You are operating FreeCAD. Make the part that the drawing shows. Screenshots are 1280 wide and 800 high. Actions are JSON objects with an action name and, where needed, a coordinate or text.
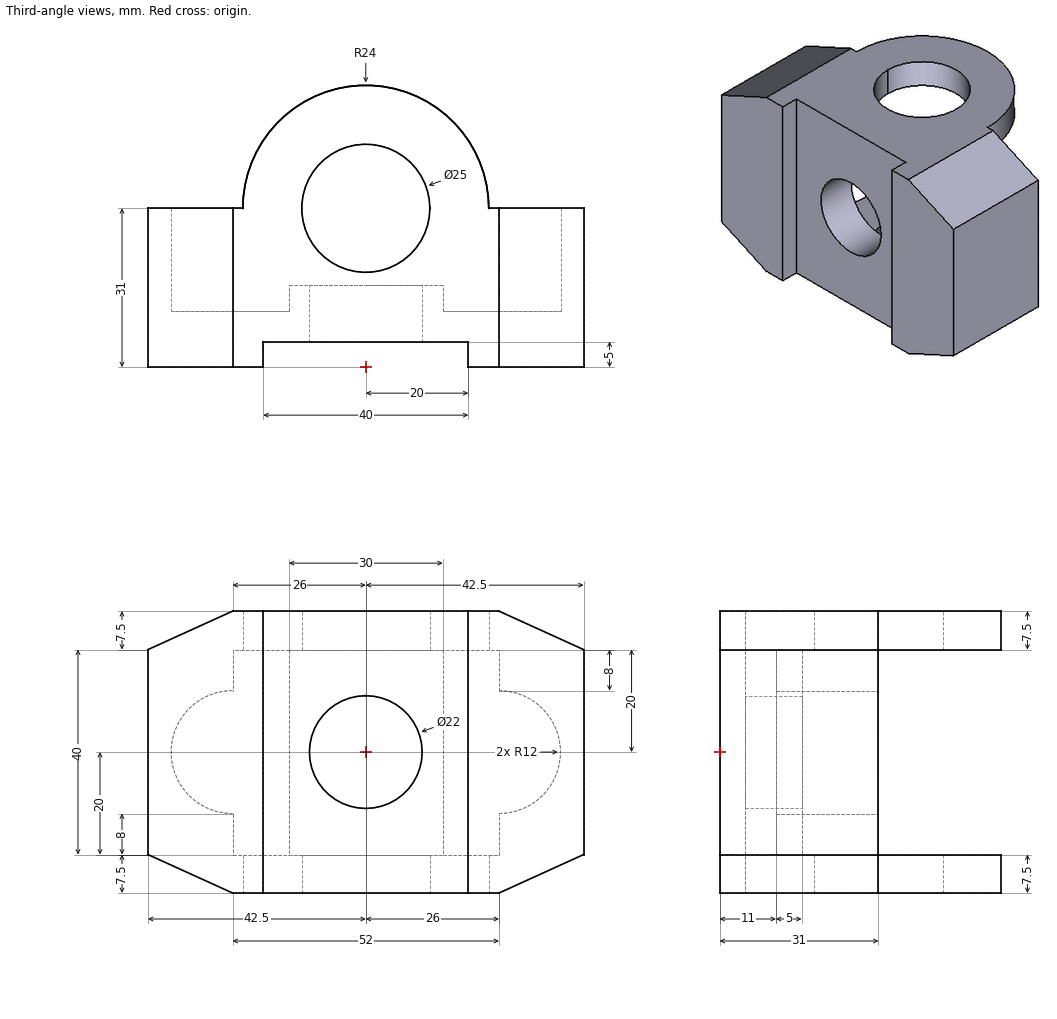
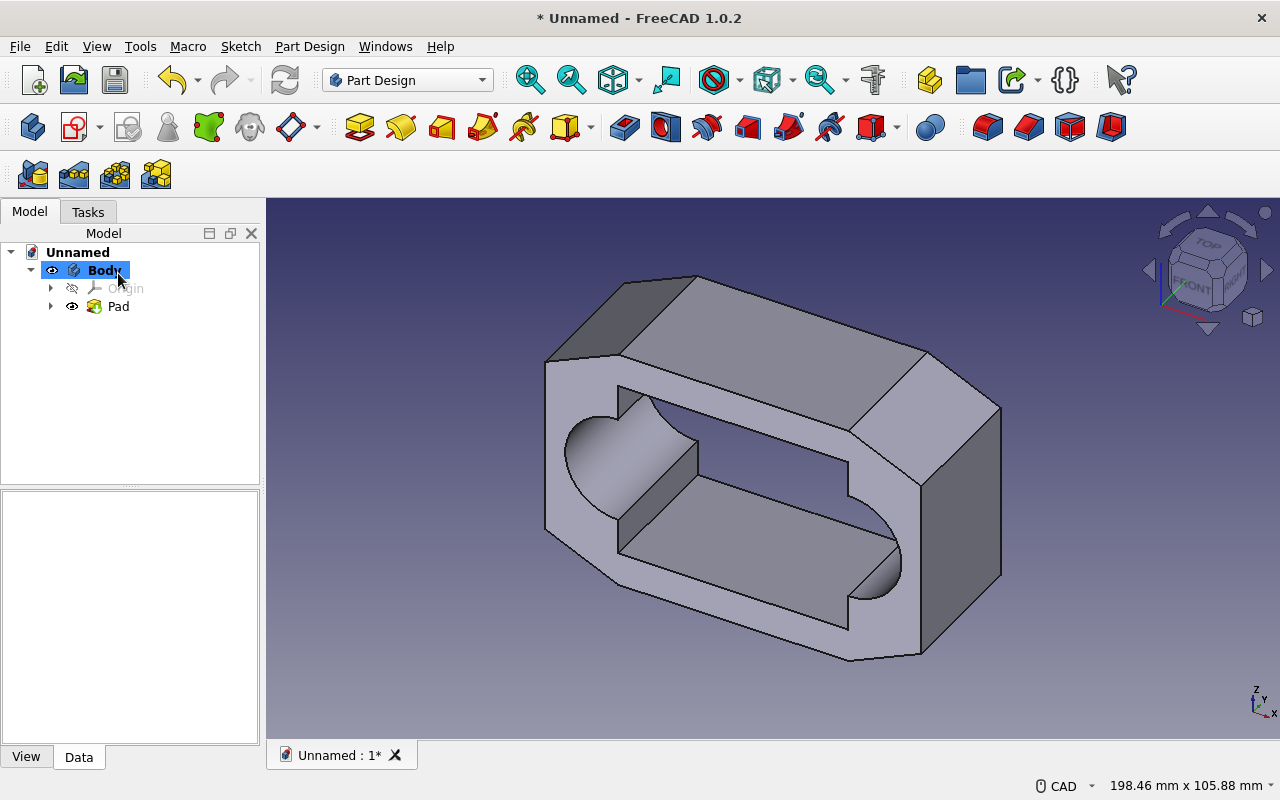
{"action": "left_click", "coordinate": [806, 363]}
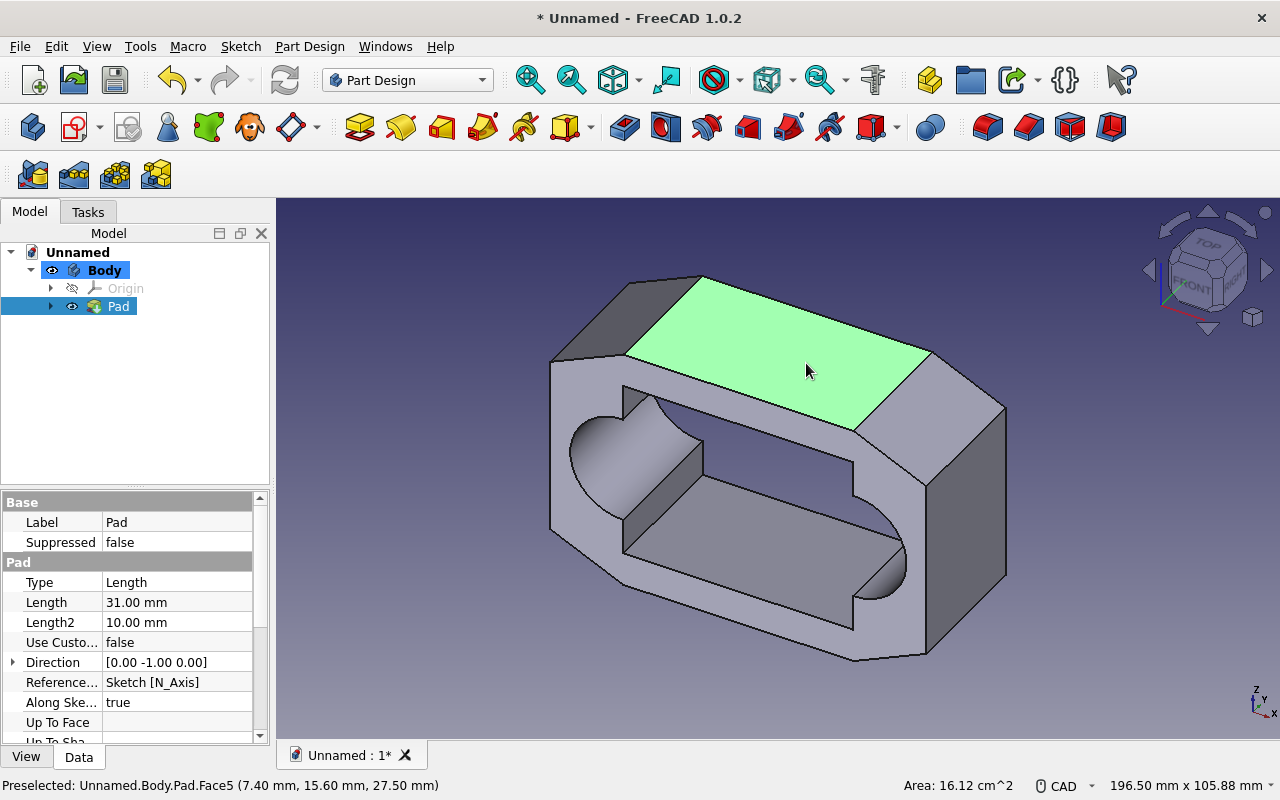
{"action": "left_click", "coordinate": [74, 128]}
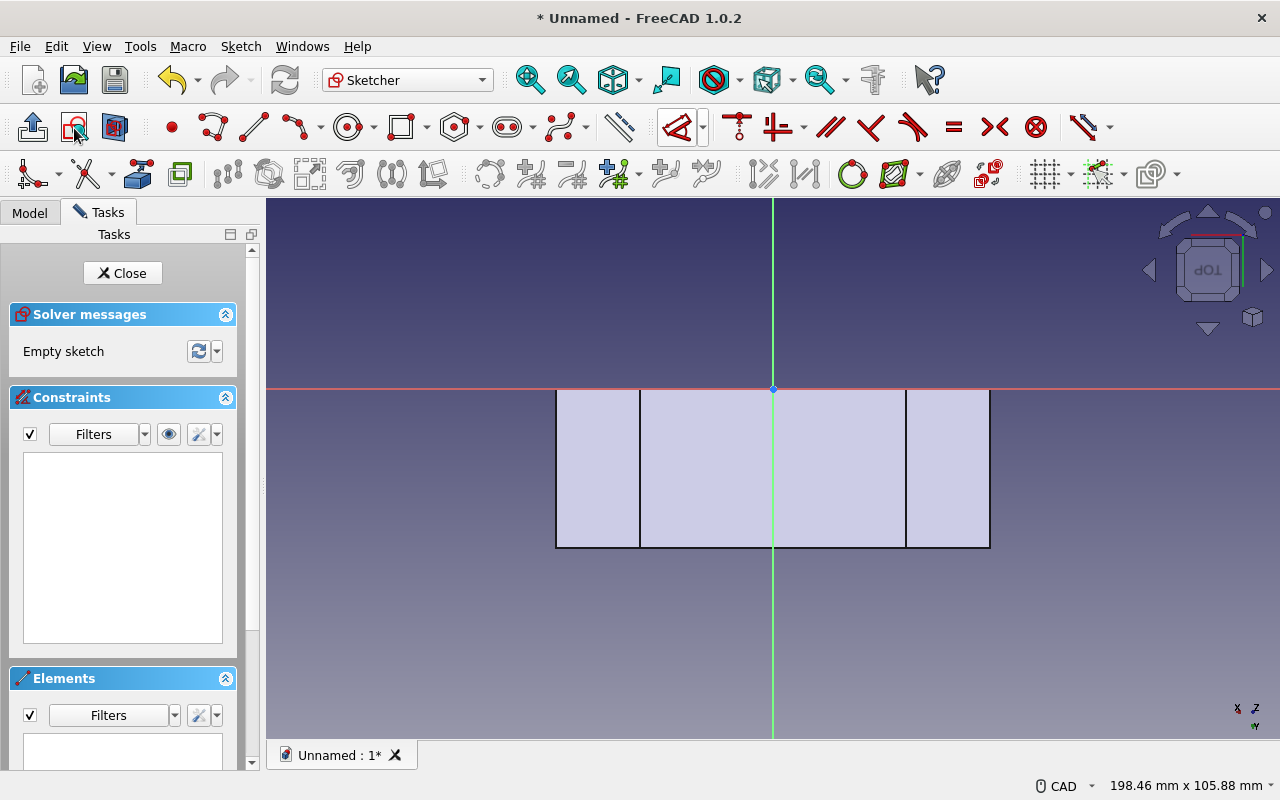
{"action": "left_click", "coordinate": [254, 128]}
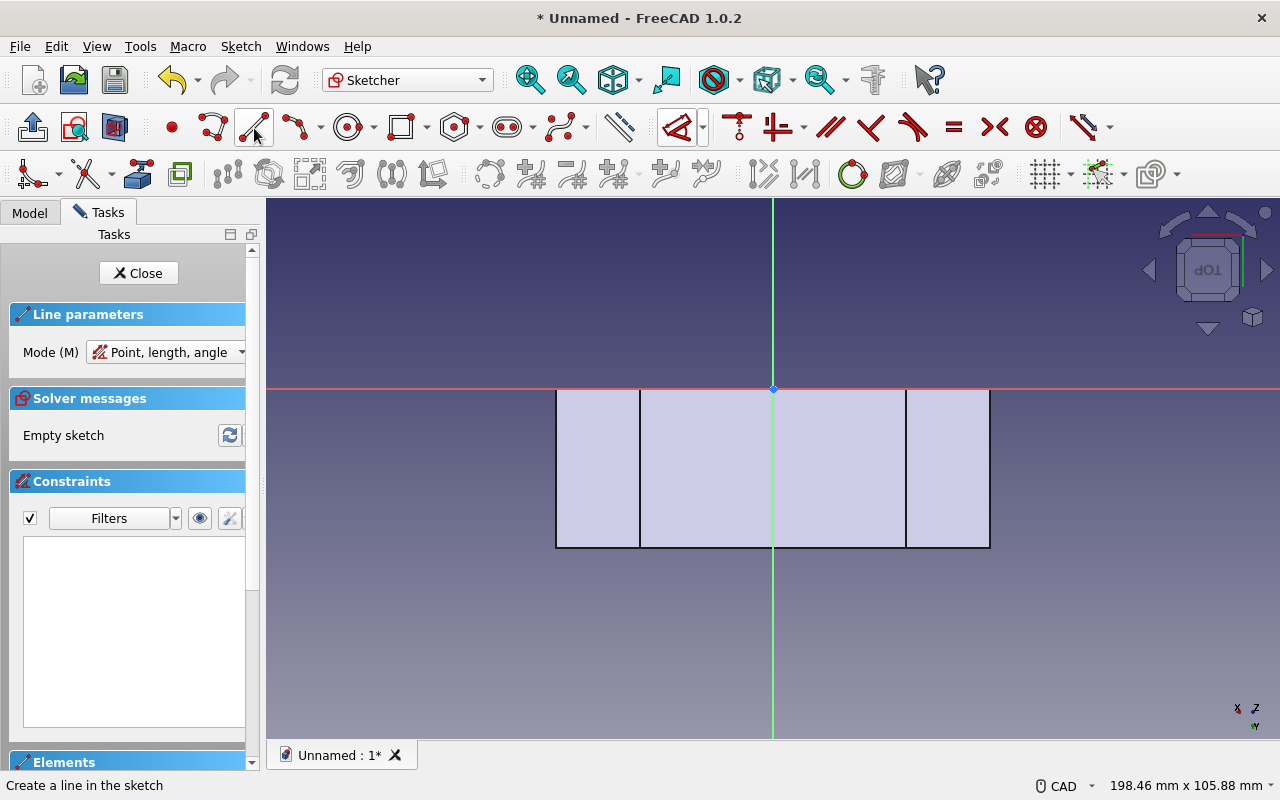
{"action": "left_click", "coordinate": [896, 548]}
{"action": "left_click", "coordinate": [650, 548]}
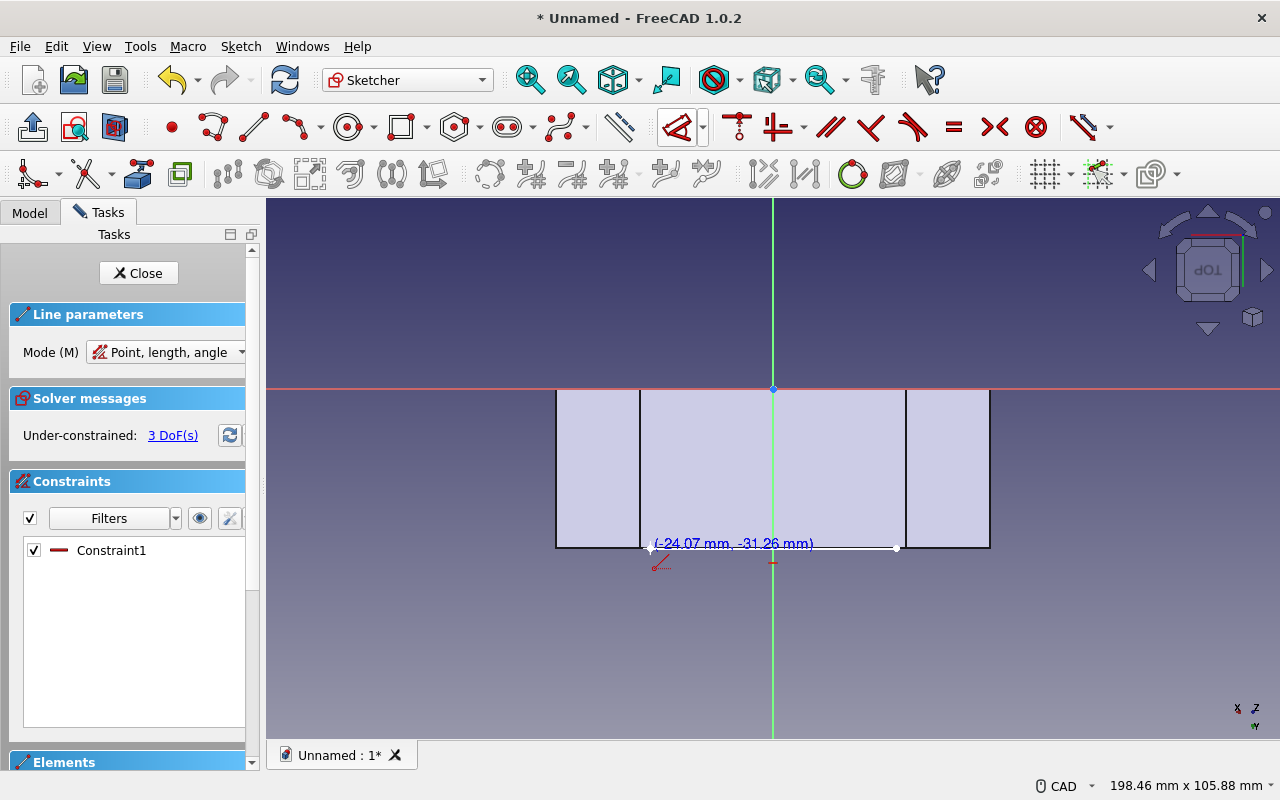
{"action": "left_click", "coordinate": [294, 128]}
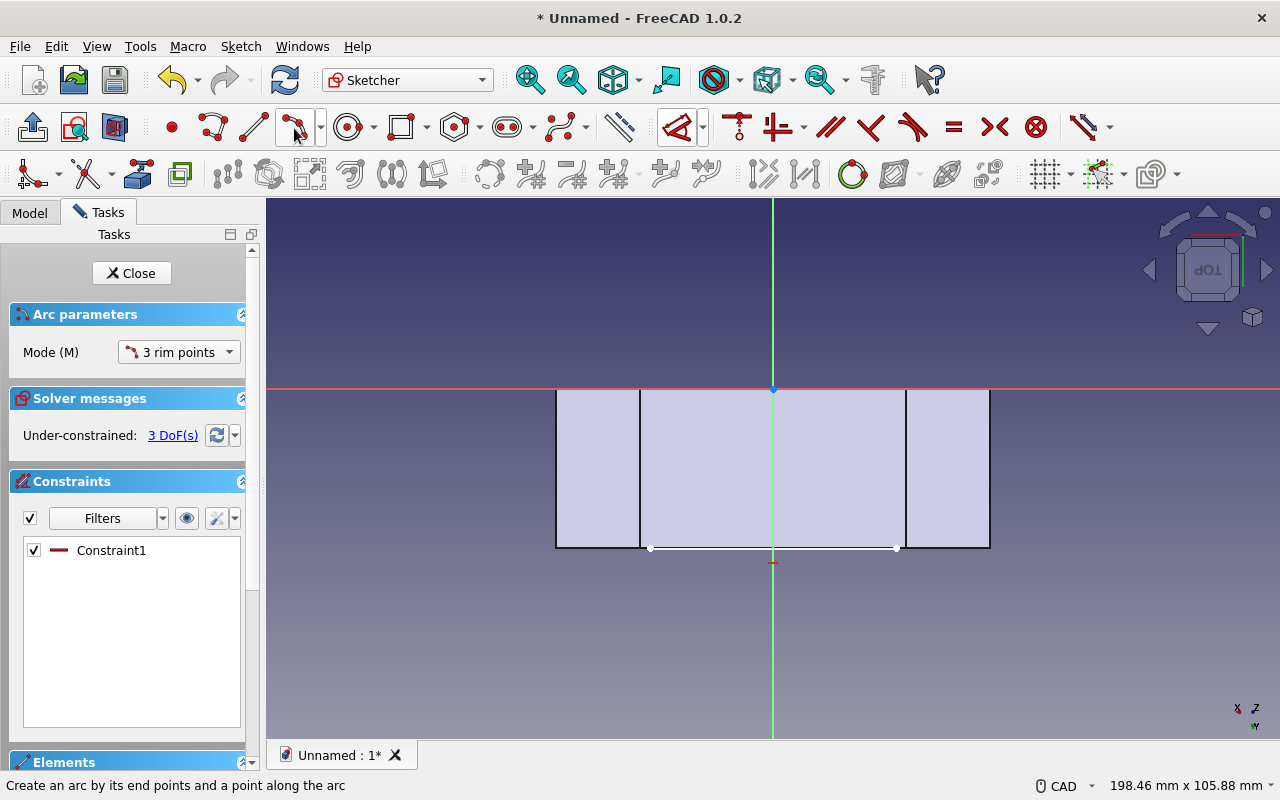
{"action": "left_click", "coordinate": [650, 549]}
{"action": "left_click", "coordinate": [896, 549]}
{"action": "left_click", "coordinate": [735, 664]}
{"action": "key", "text": "Escape"}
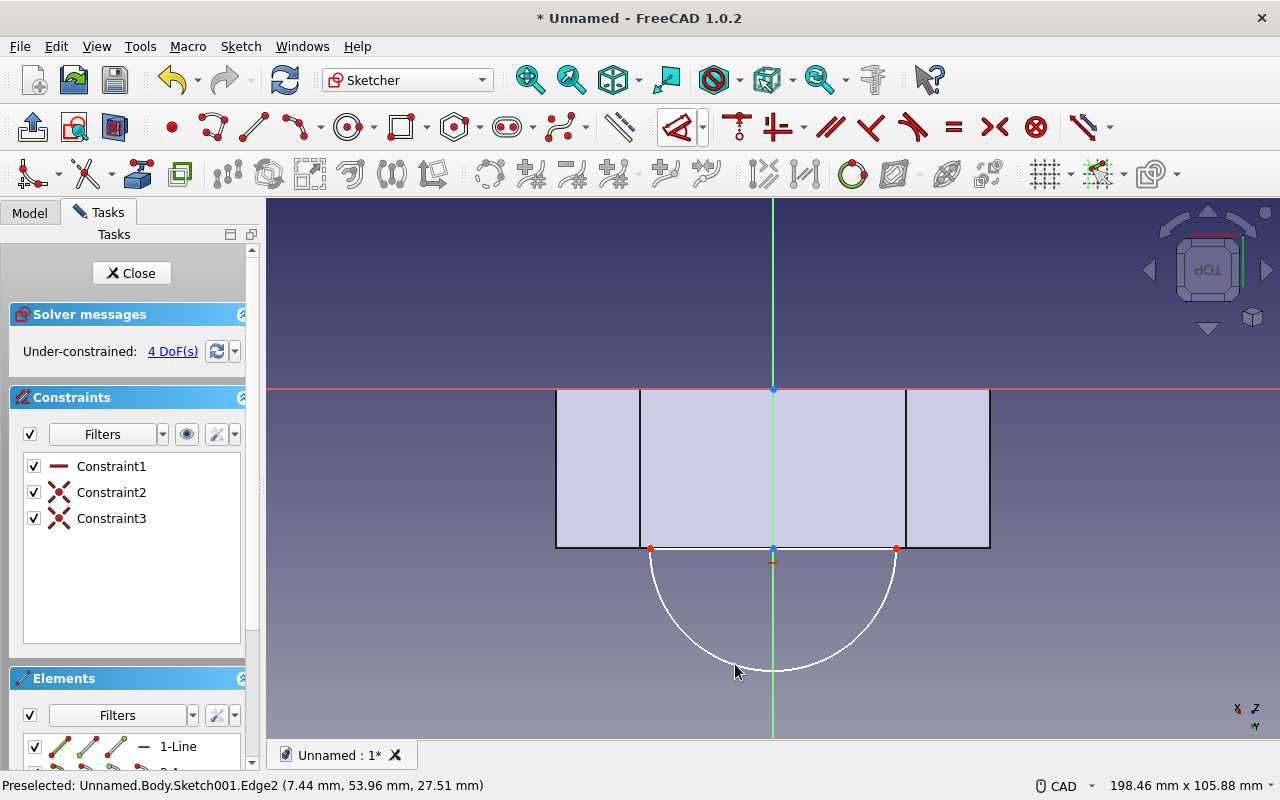
{"action": "left_click", "coordinate": [773, 548]}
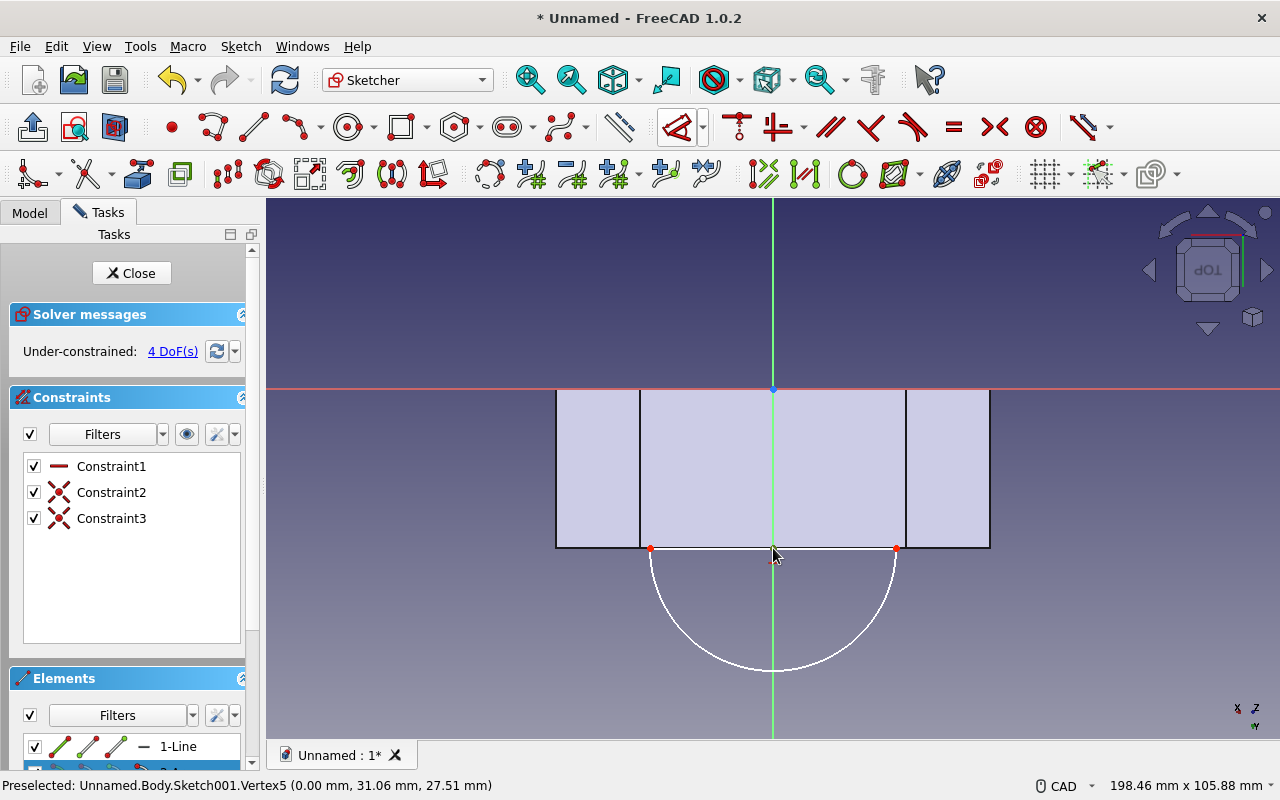
{"action": "left_click", "coordinate": [773, 607]}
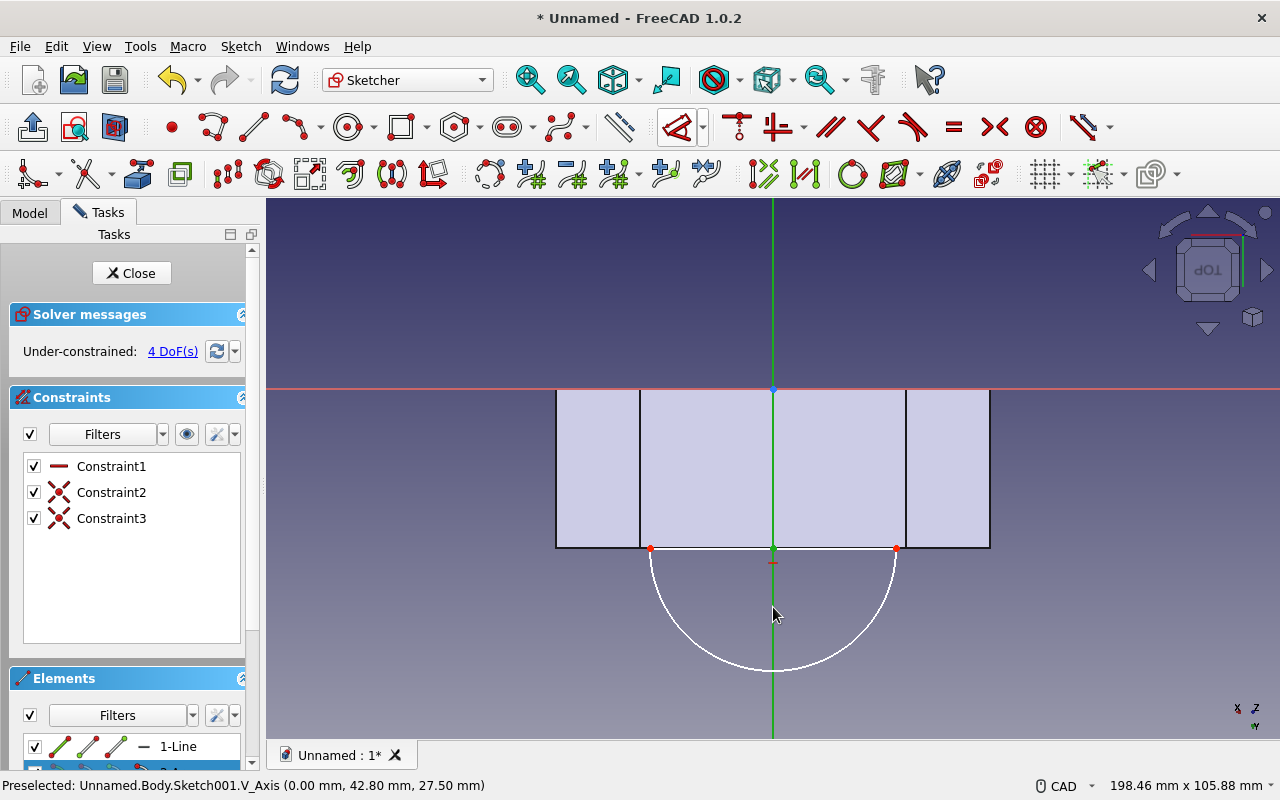
{"action": "left_click", "coordinate": [737, 128]}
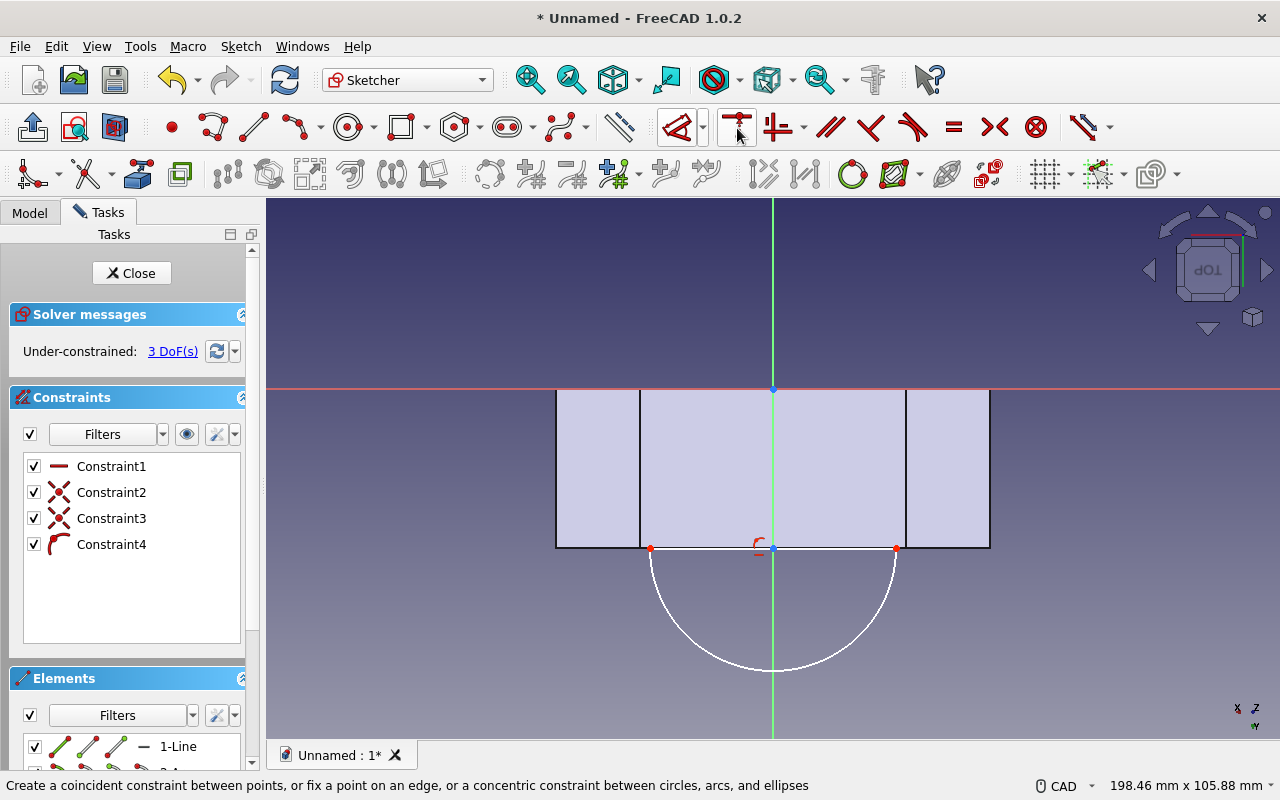
{"action": "left_click", "coordinate": [701, 648]}